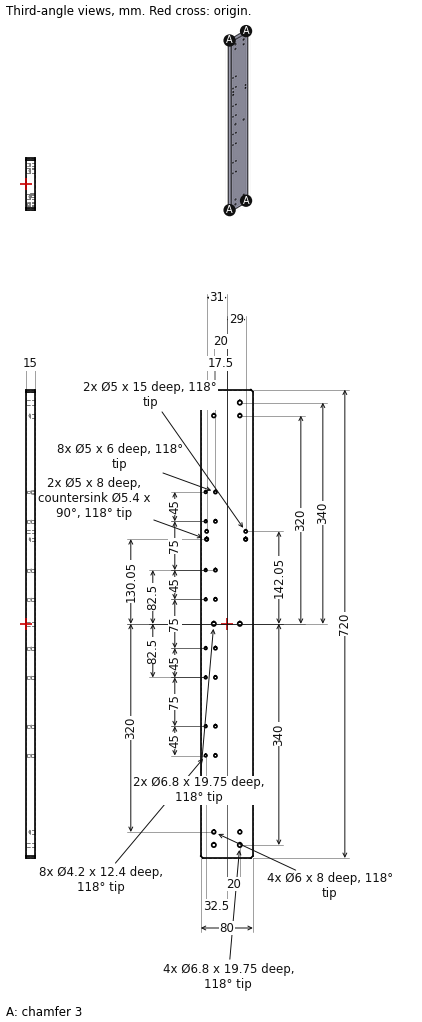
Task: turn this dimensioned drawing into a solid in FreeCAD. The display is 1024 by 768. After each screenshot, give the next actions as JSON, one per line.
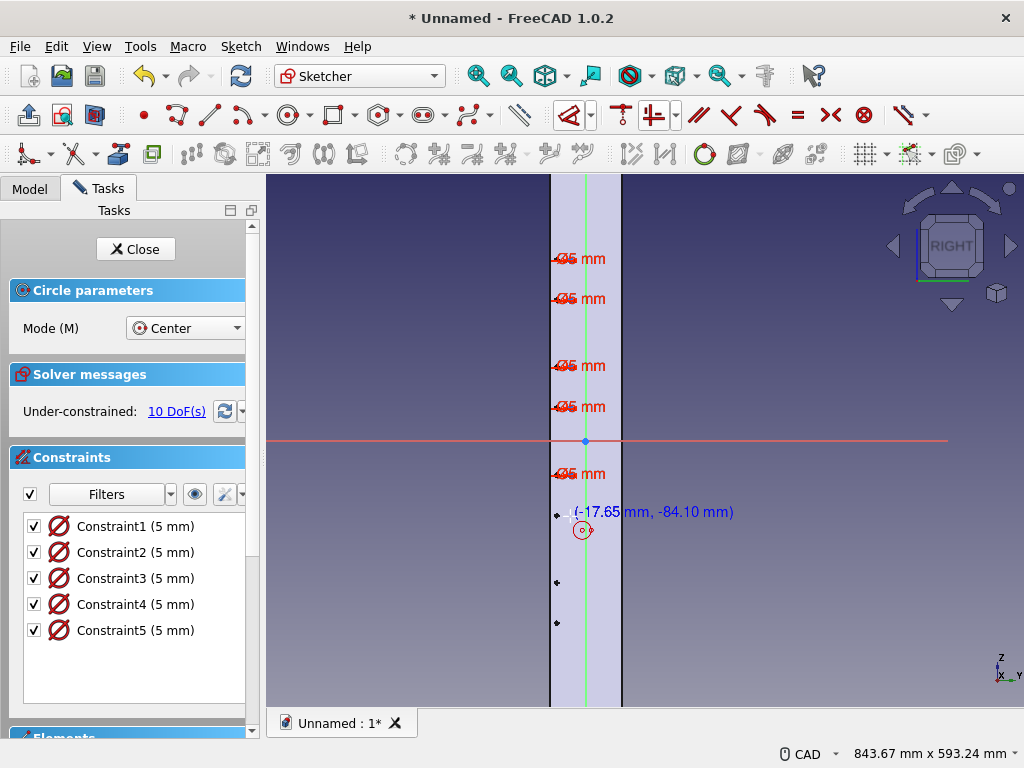
{"action": "left_click", "coordinate": [570, 516]}
{"action": "mouse_move", "coordinate": [572, 514]}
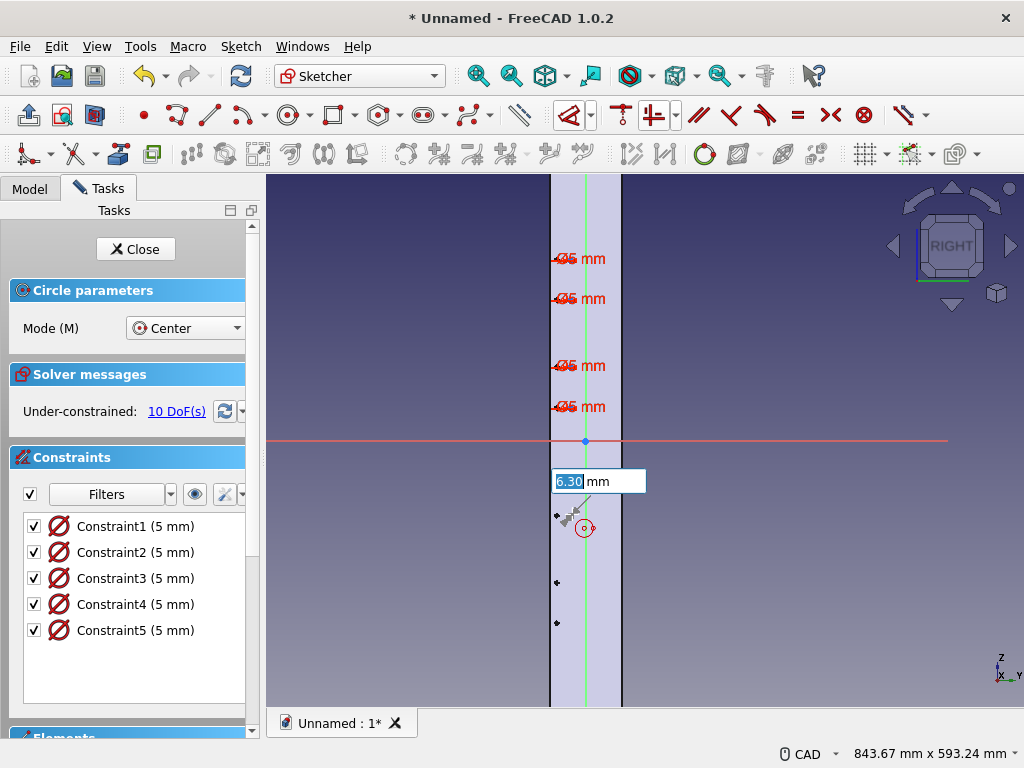
{"action": "type", "text": "5"}
{"action": "key", "text": "Return"}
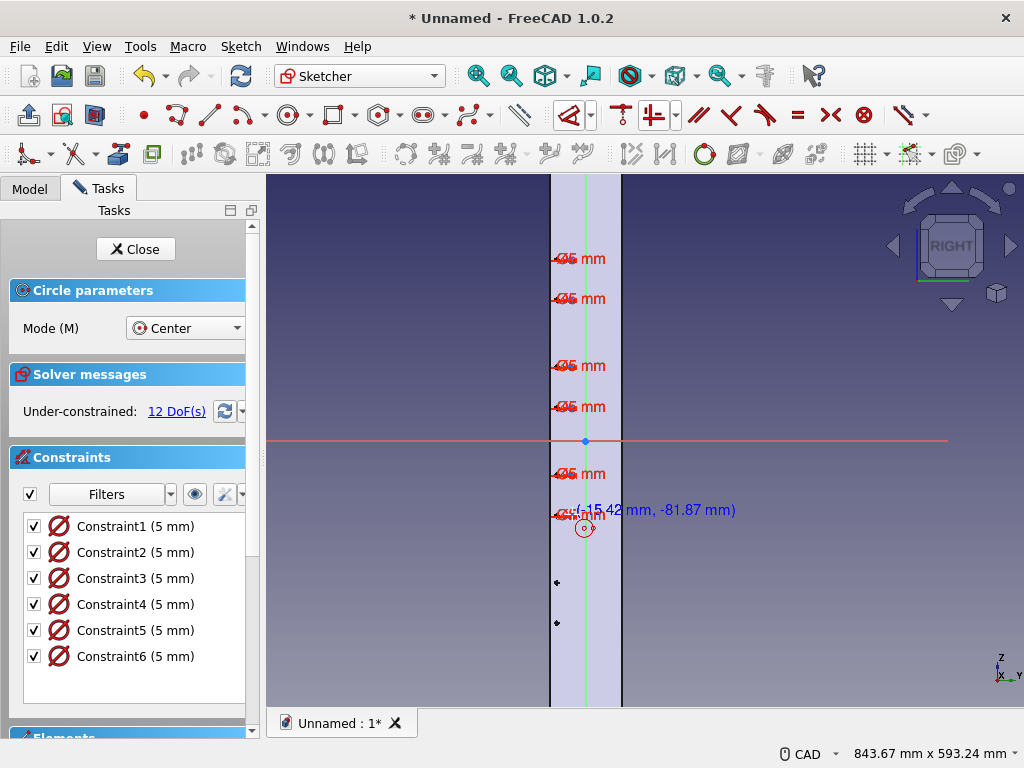
{"action": "scroll", "coordinate": [570, 583], "scroll_direction": "up", "scroll_amount": 12}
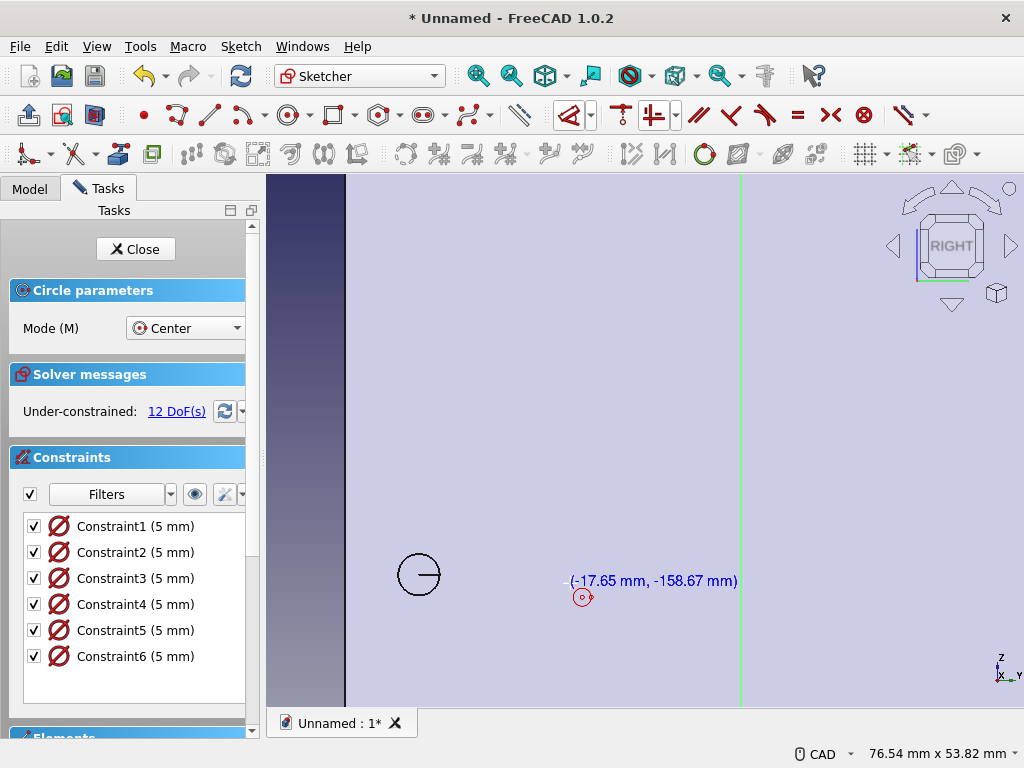
{"action": "scroll", "coordinate": [570, 583], "scroll_direction": "down", "scroll_amount": 12}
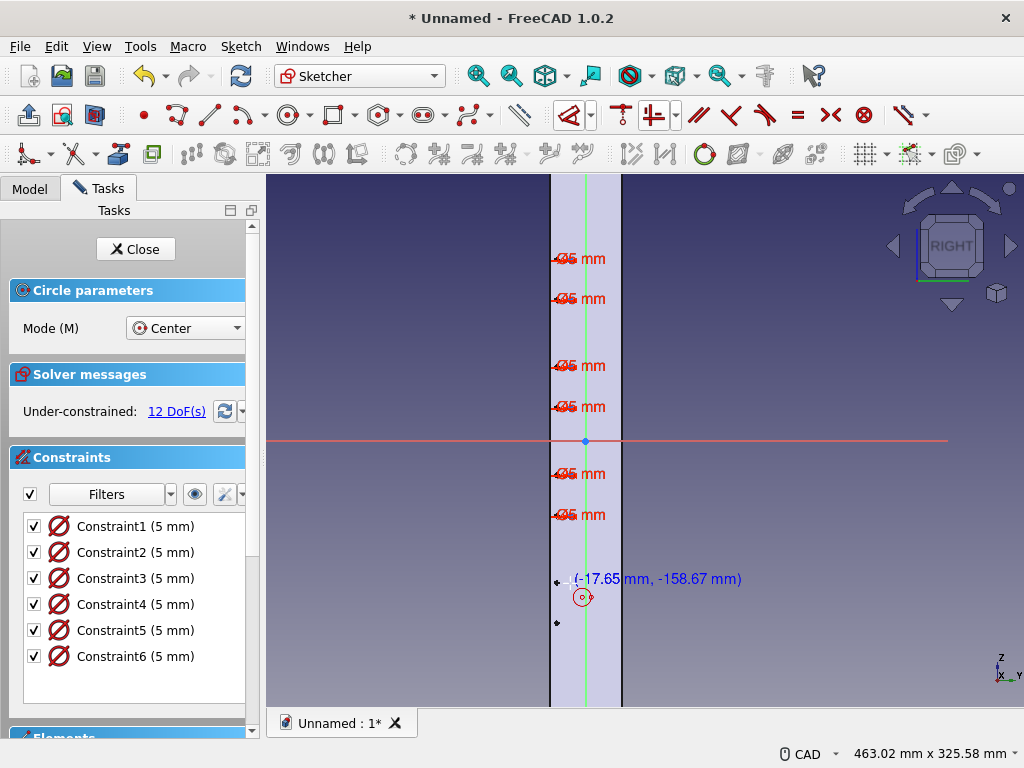
{"action": "left_click", "coordinate": [570, 583]}
{"action": "mouse_move", "coordinate": [572, 581]}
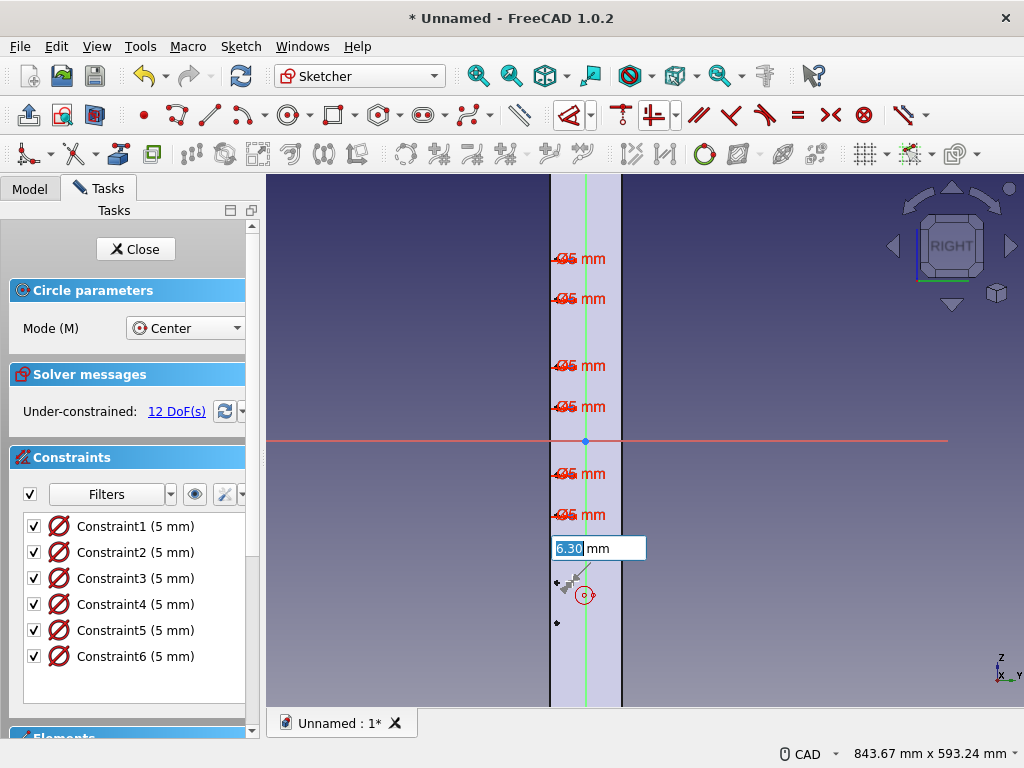
{"action": "type", "text": "5"}
{"action": "key", "text": "Return"}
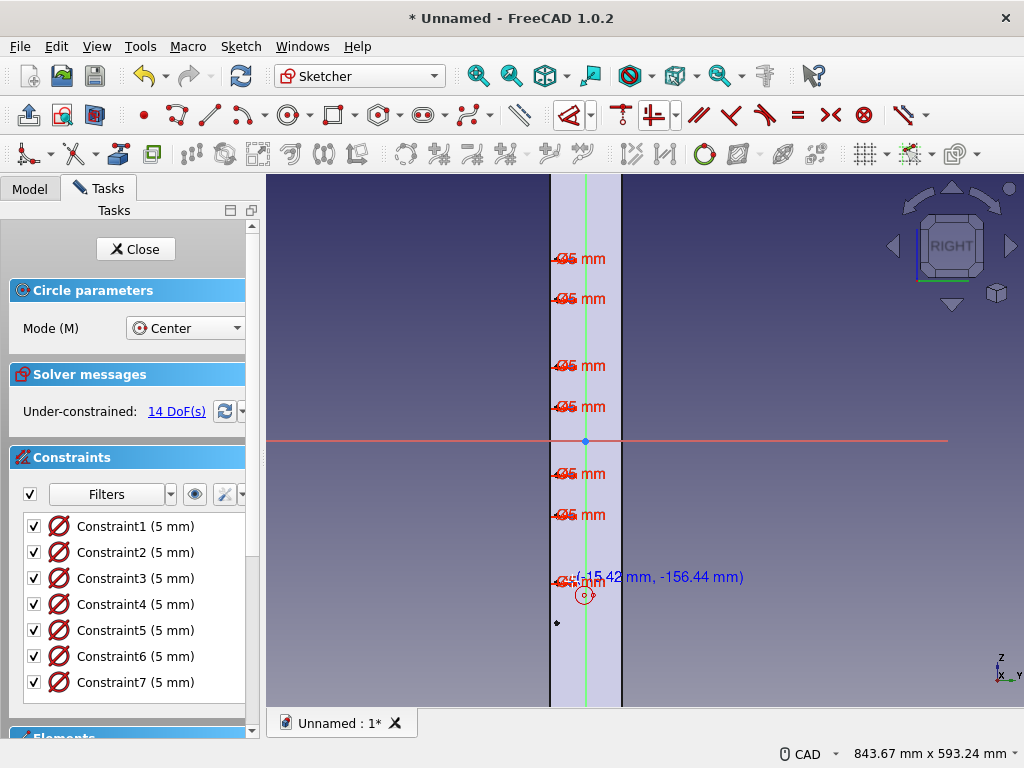
{"action": "scroll", "coordinate": [570, 623], "scroll_direction": "up", "scroll_amount": 12}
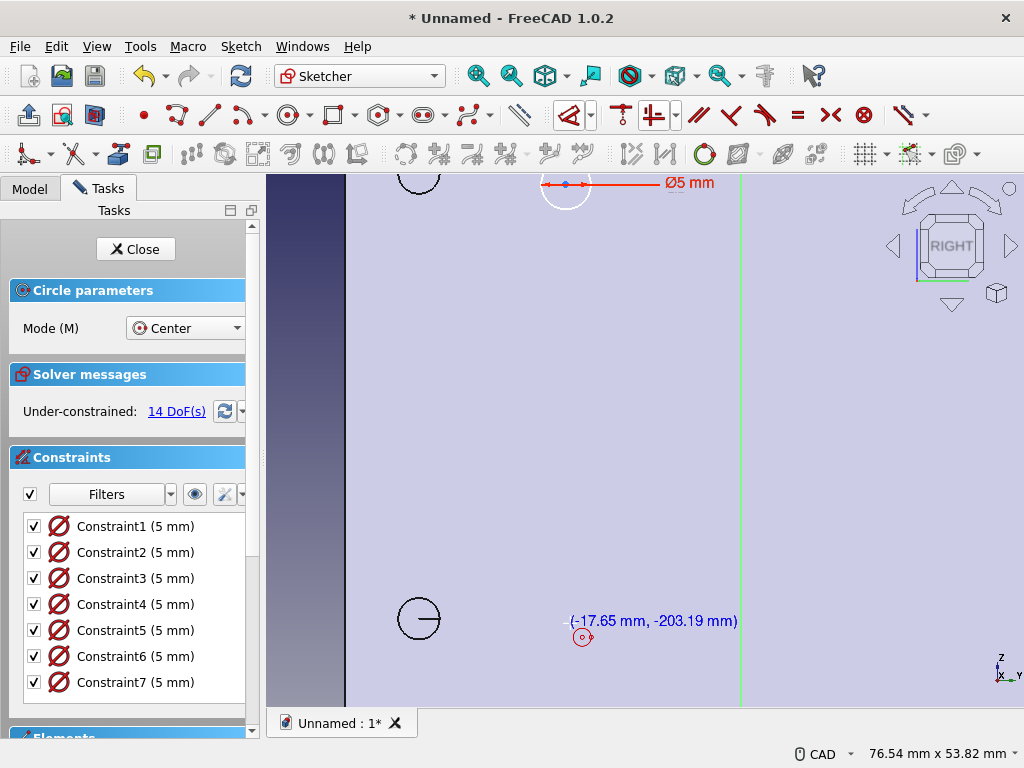
{"action": "scroll", "coordinate": [570, 623], "scroll_direction": "down", "scroll_amount": 12}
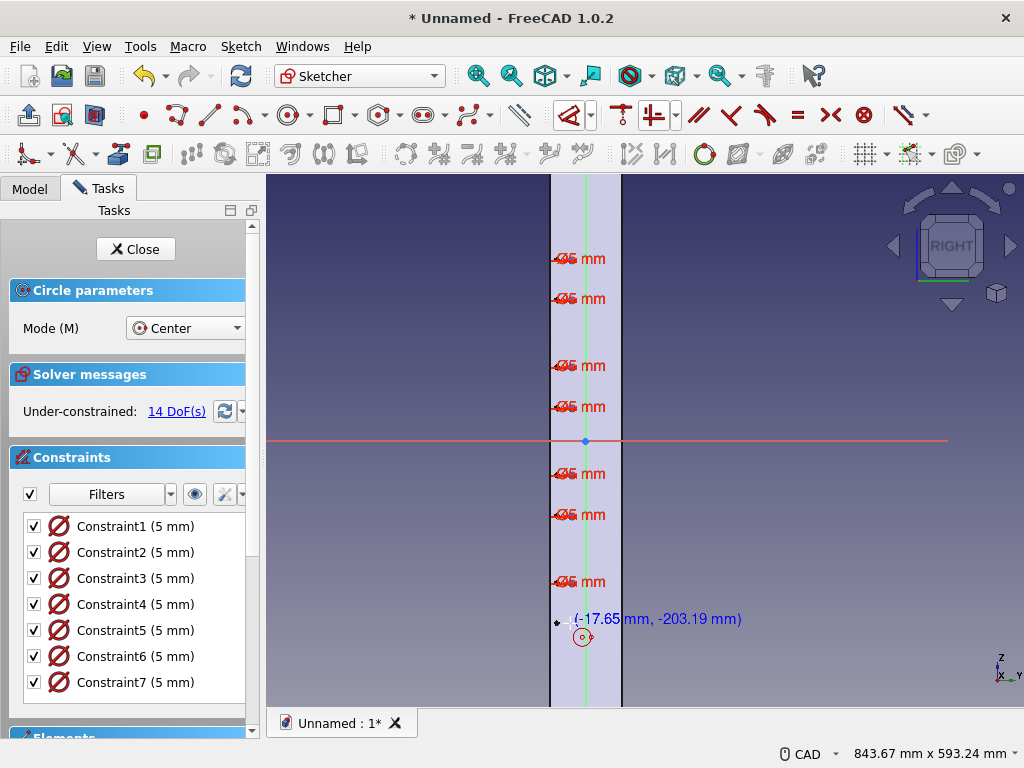
{"action": "left_click", "coordinate": [570, 623]}
{"action": "mouse_move", "coordinate": [572, 622]}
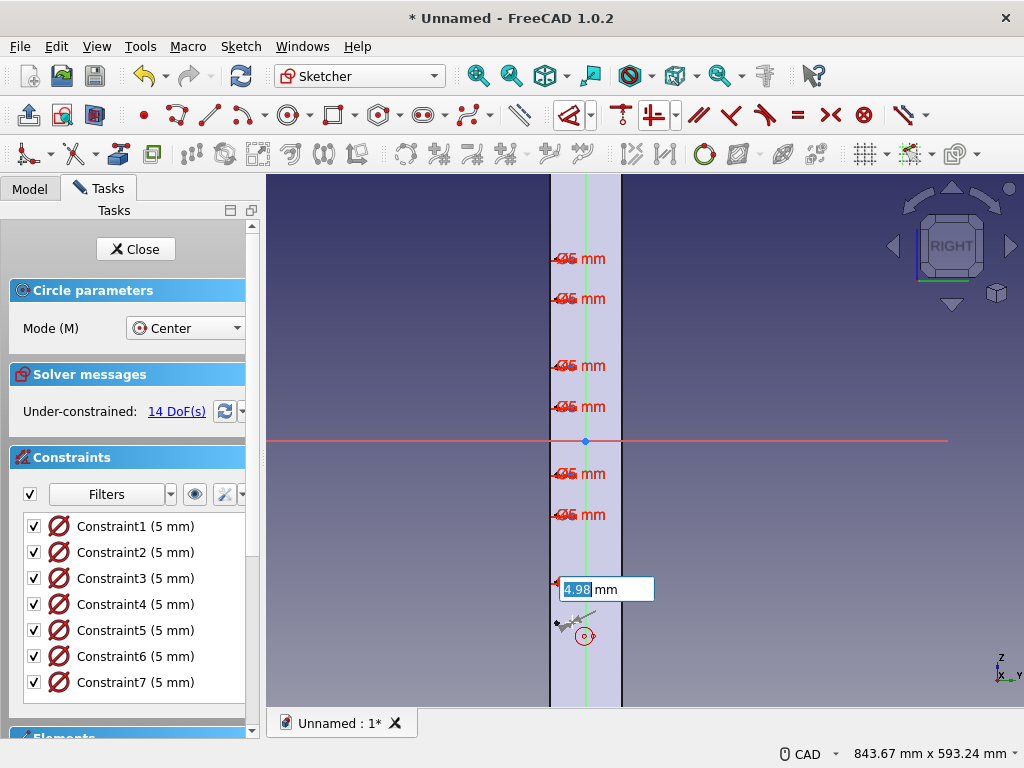
{"action": "type", "text": "5"}
{"action": "key", "text": "Return"}
{"action": "key", "text": "Escape"}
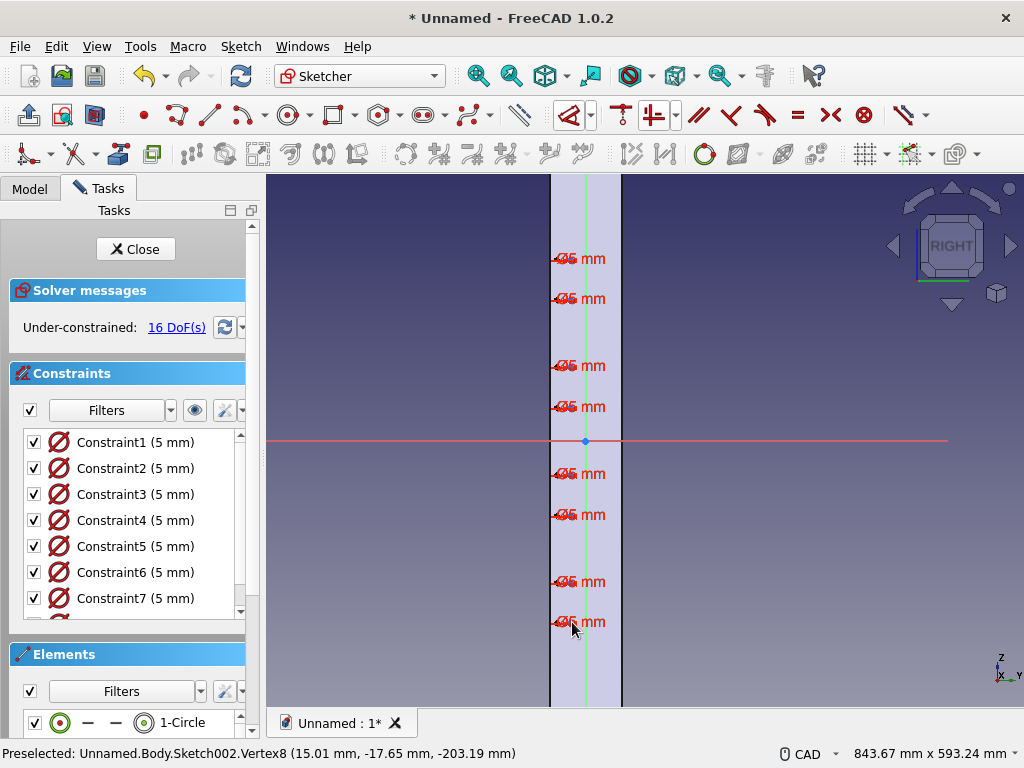
{"action": "left_click", "coordinate": [570, 261]}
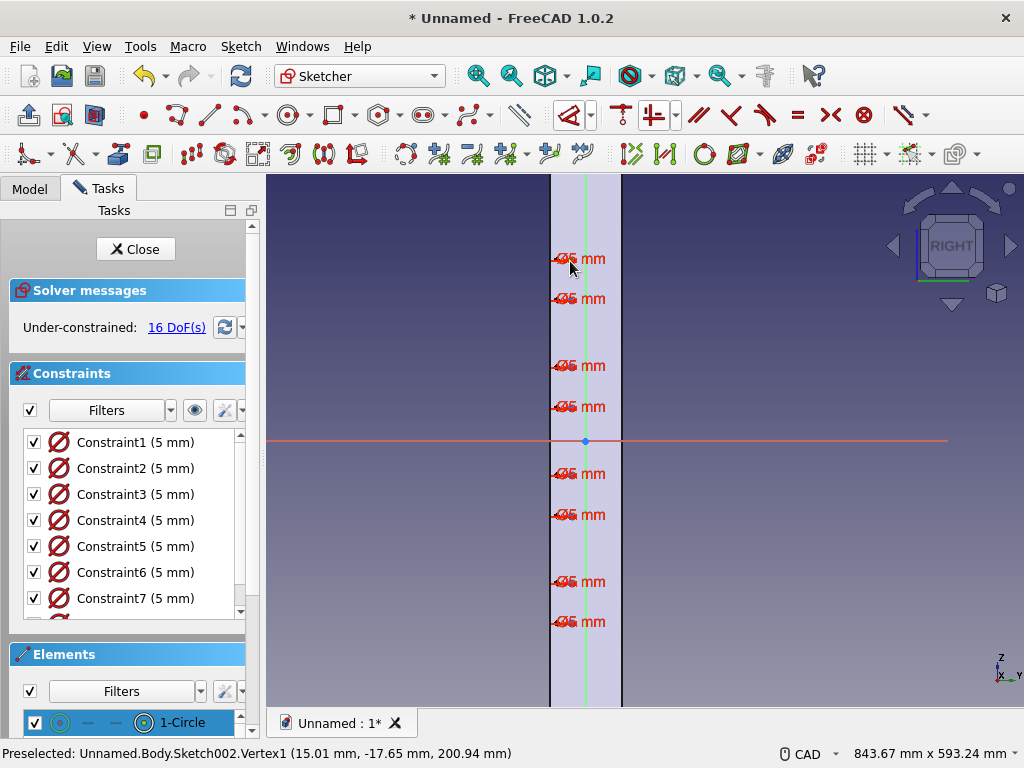
{"action": "left_click", "coordinate": [570, 301]}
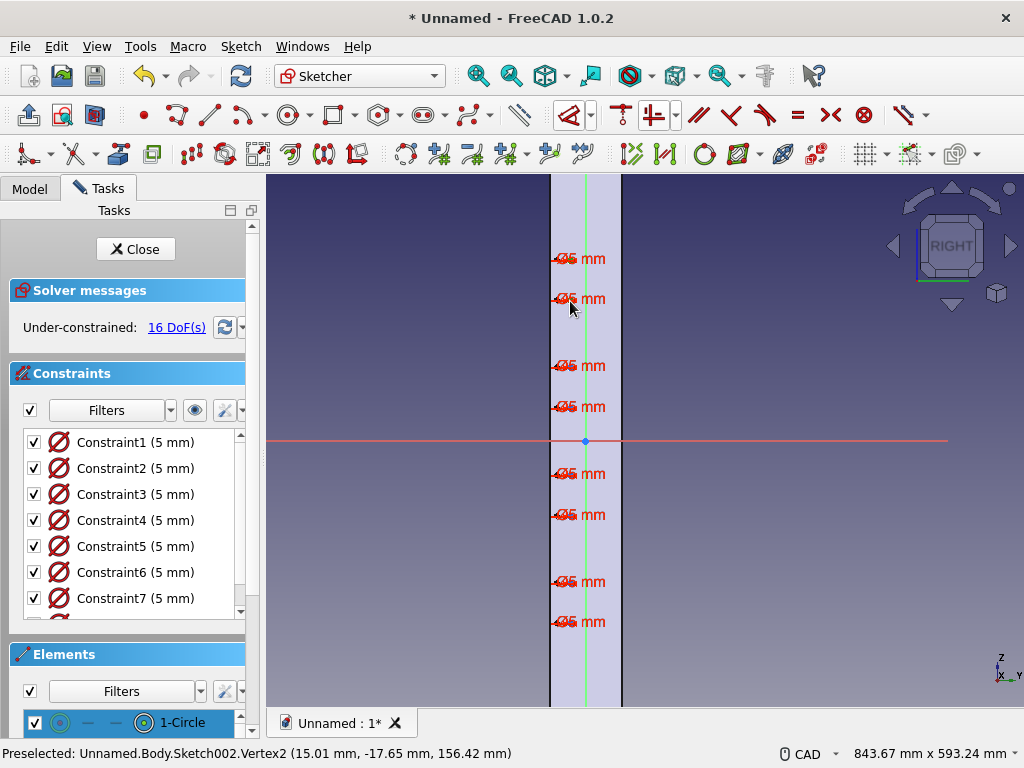
{"action": "key", "text": "v"}